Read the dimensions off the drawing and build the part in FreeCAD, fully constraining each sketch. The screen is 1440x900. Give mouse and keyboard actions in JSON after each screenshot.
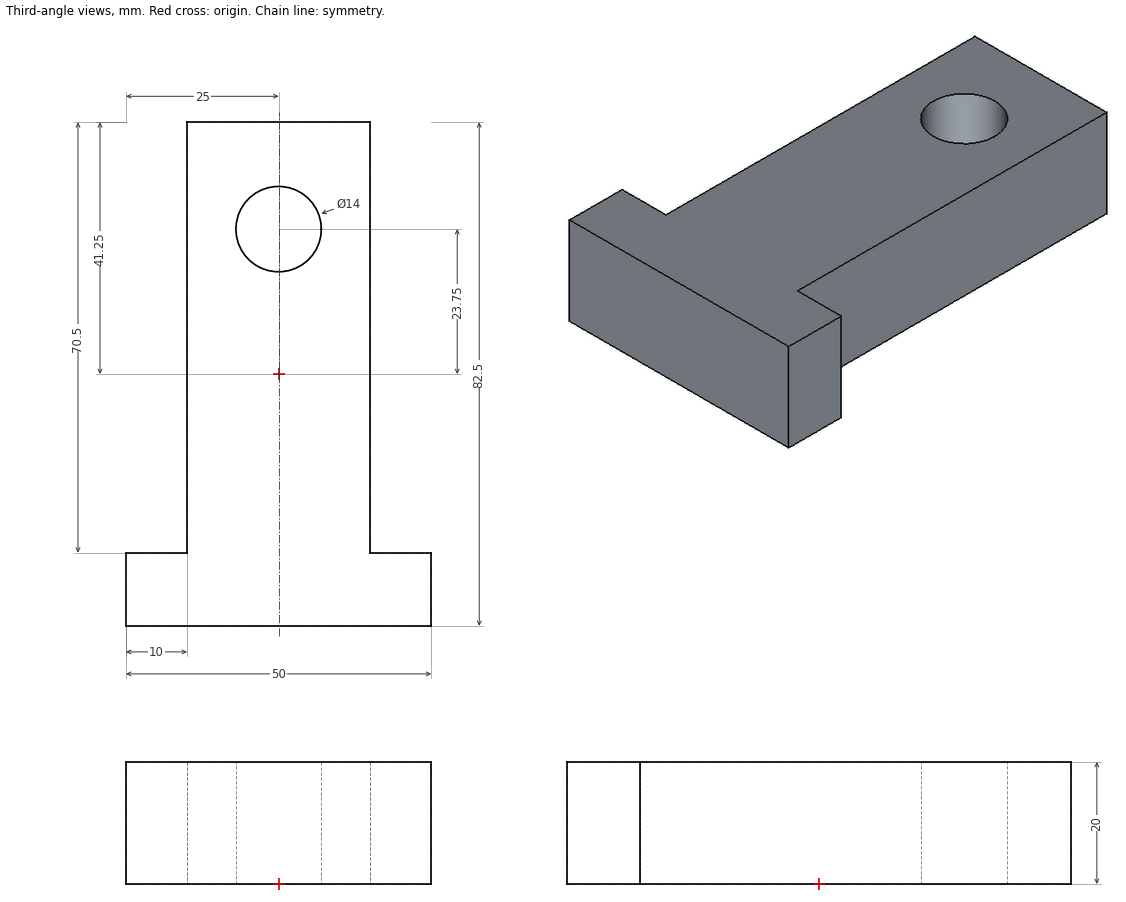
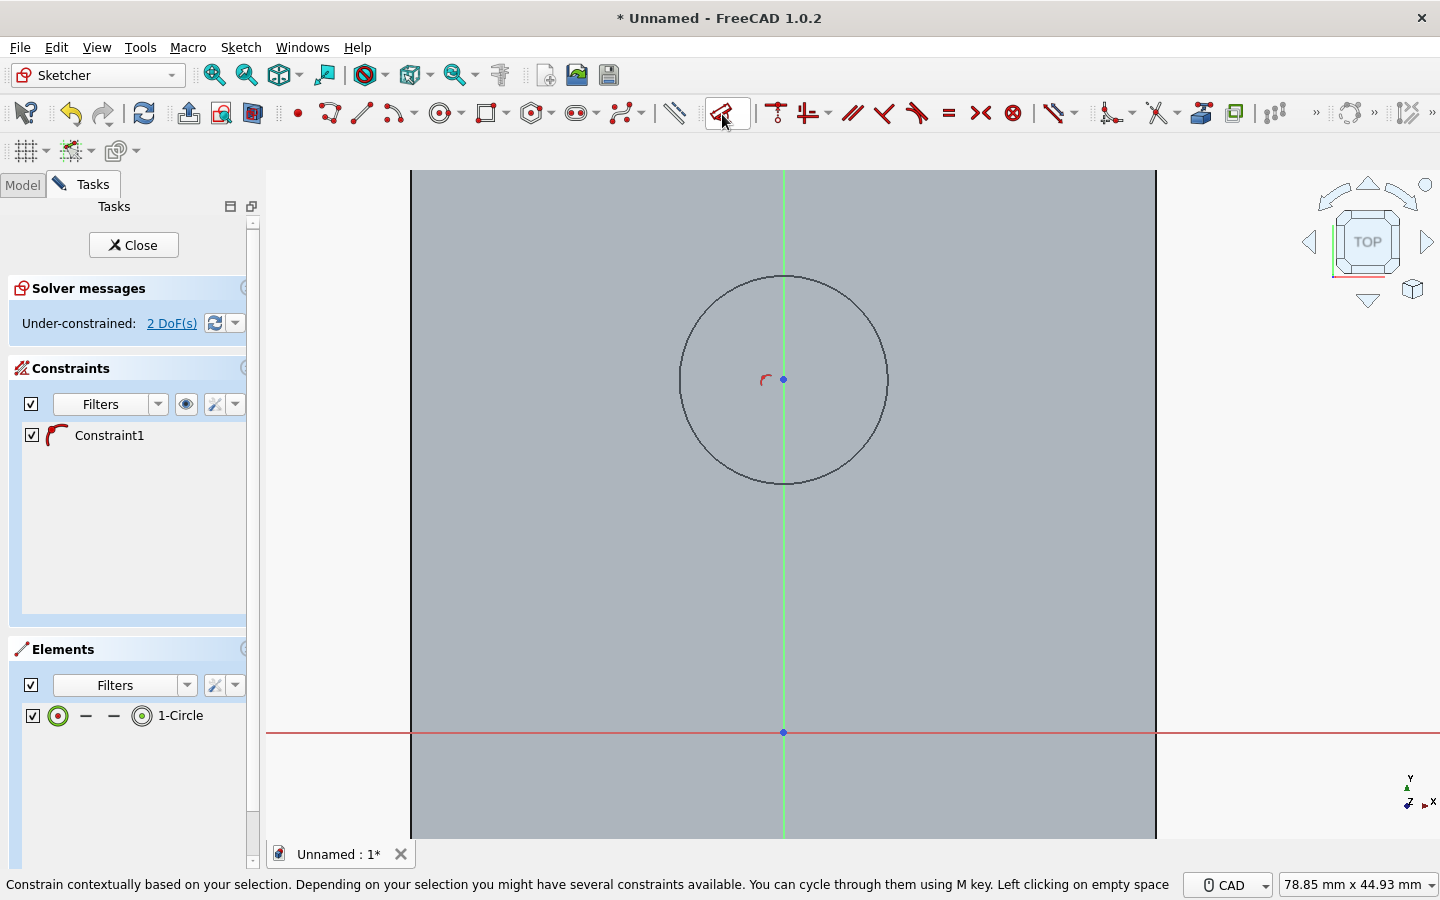
{"action": "left_click", "coordinate": [857, 306]}
{"action": "left_click", "coordinate": [880, 283]}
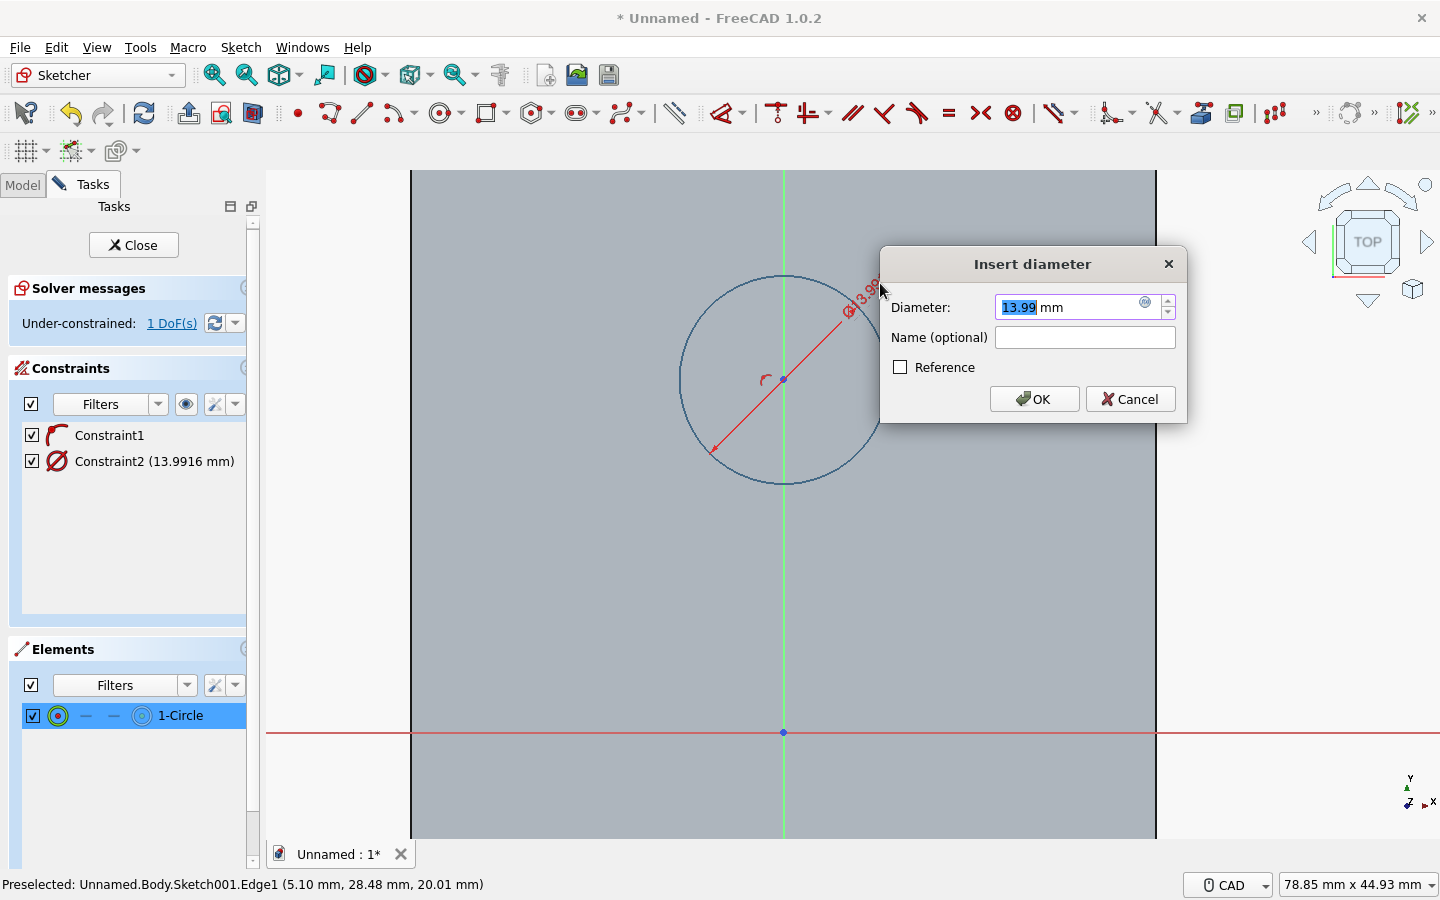
{"action": "type", "text": "14"}
{"action": "key", "text": "Return"}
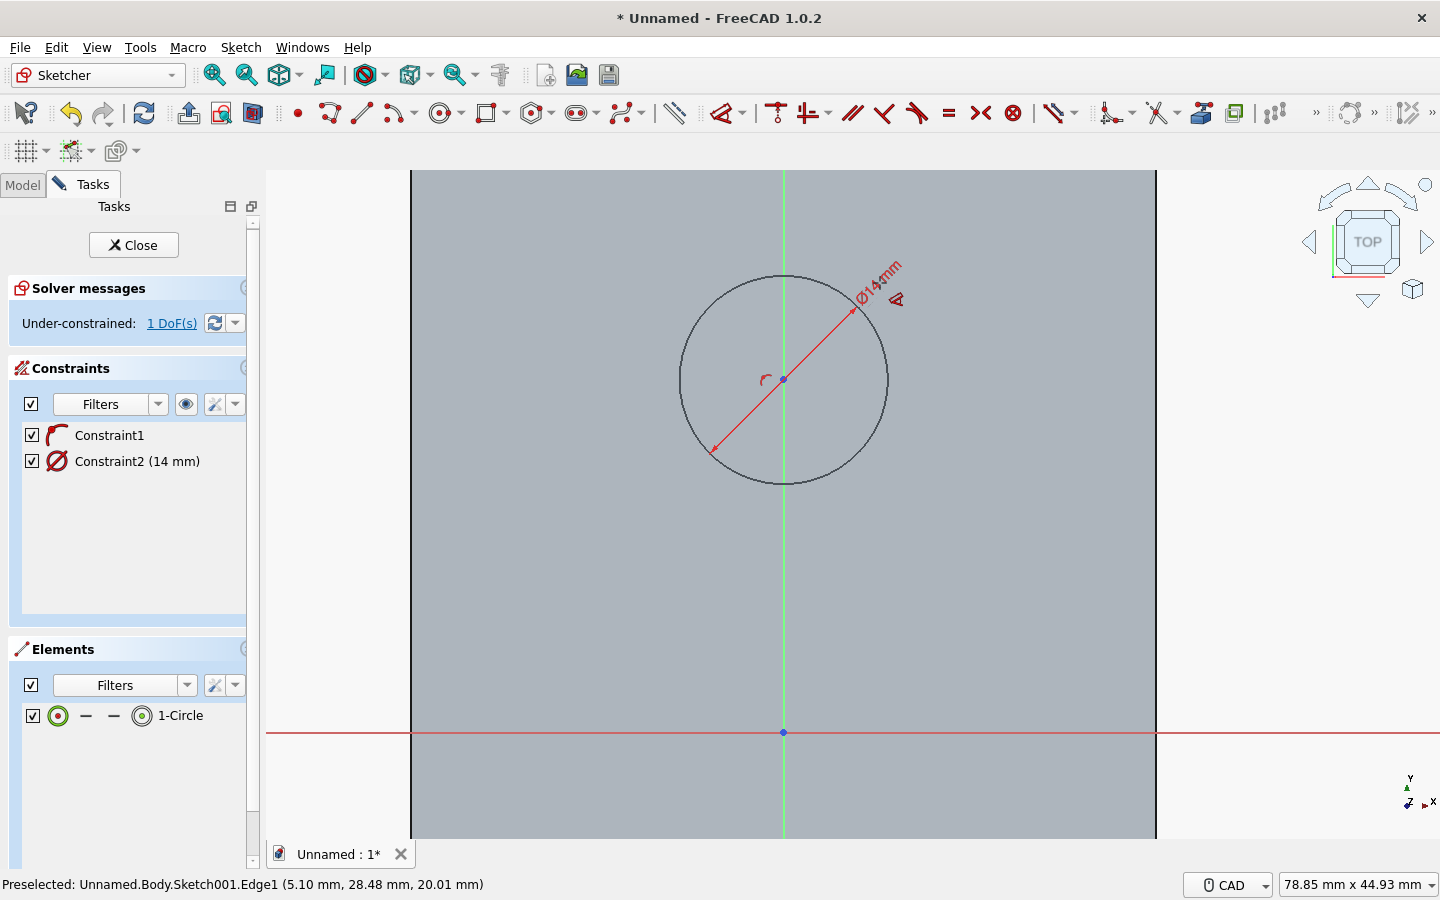
{"action": "left_click", "coordinate": [784, 380]}
{"action": "left_click", "coordinate": [818, 556]}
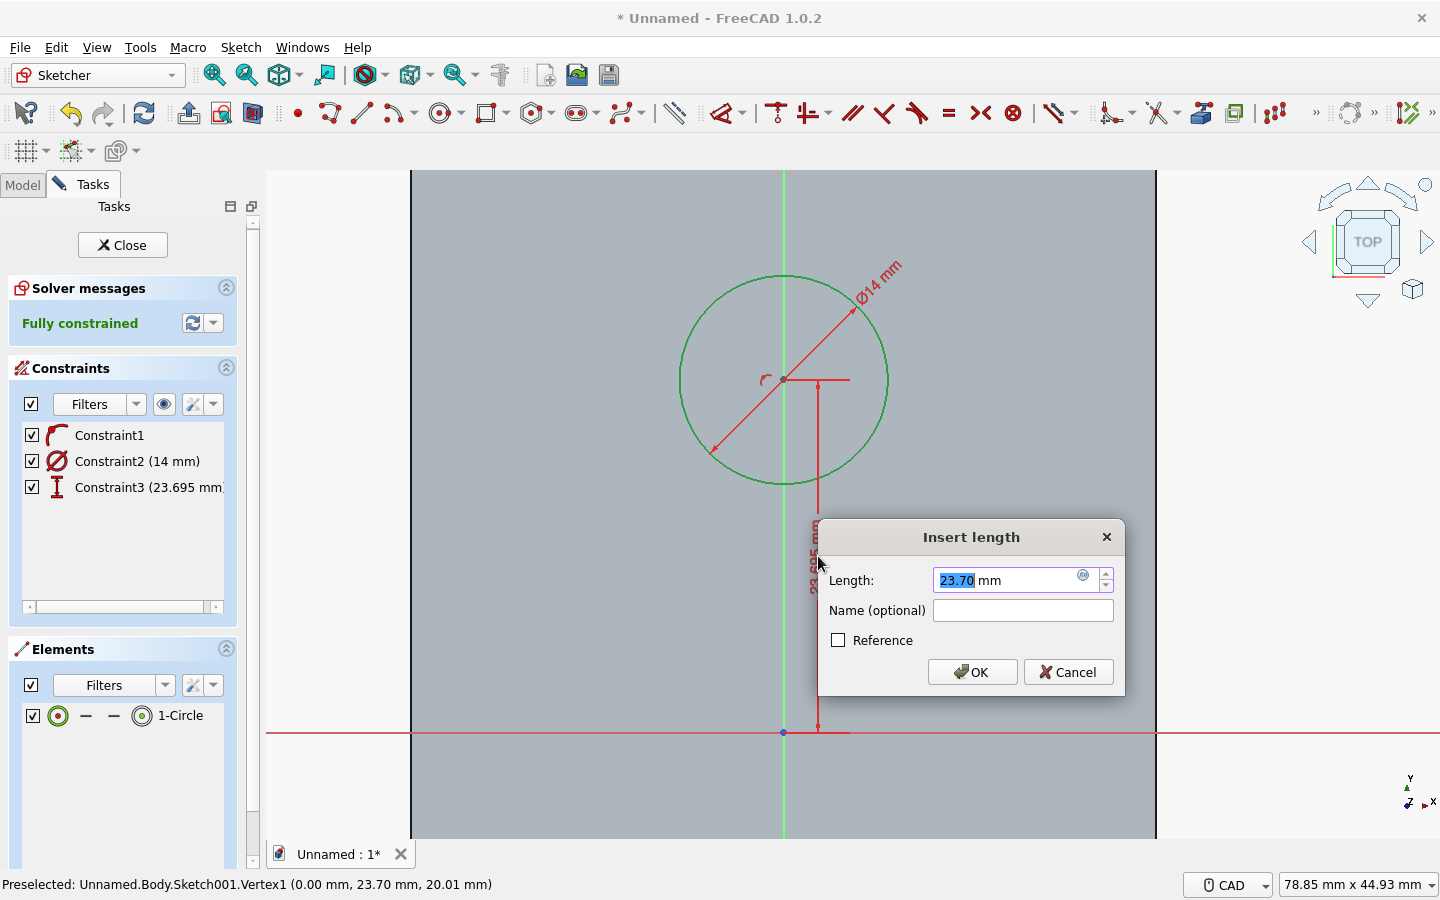
{"action": "type", "text": "23.75"}
{"action": "key", "text": "Return"}
{"action": "key", "text": "Escape"}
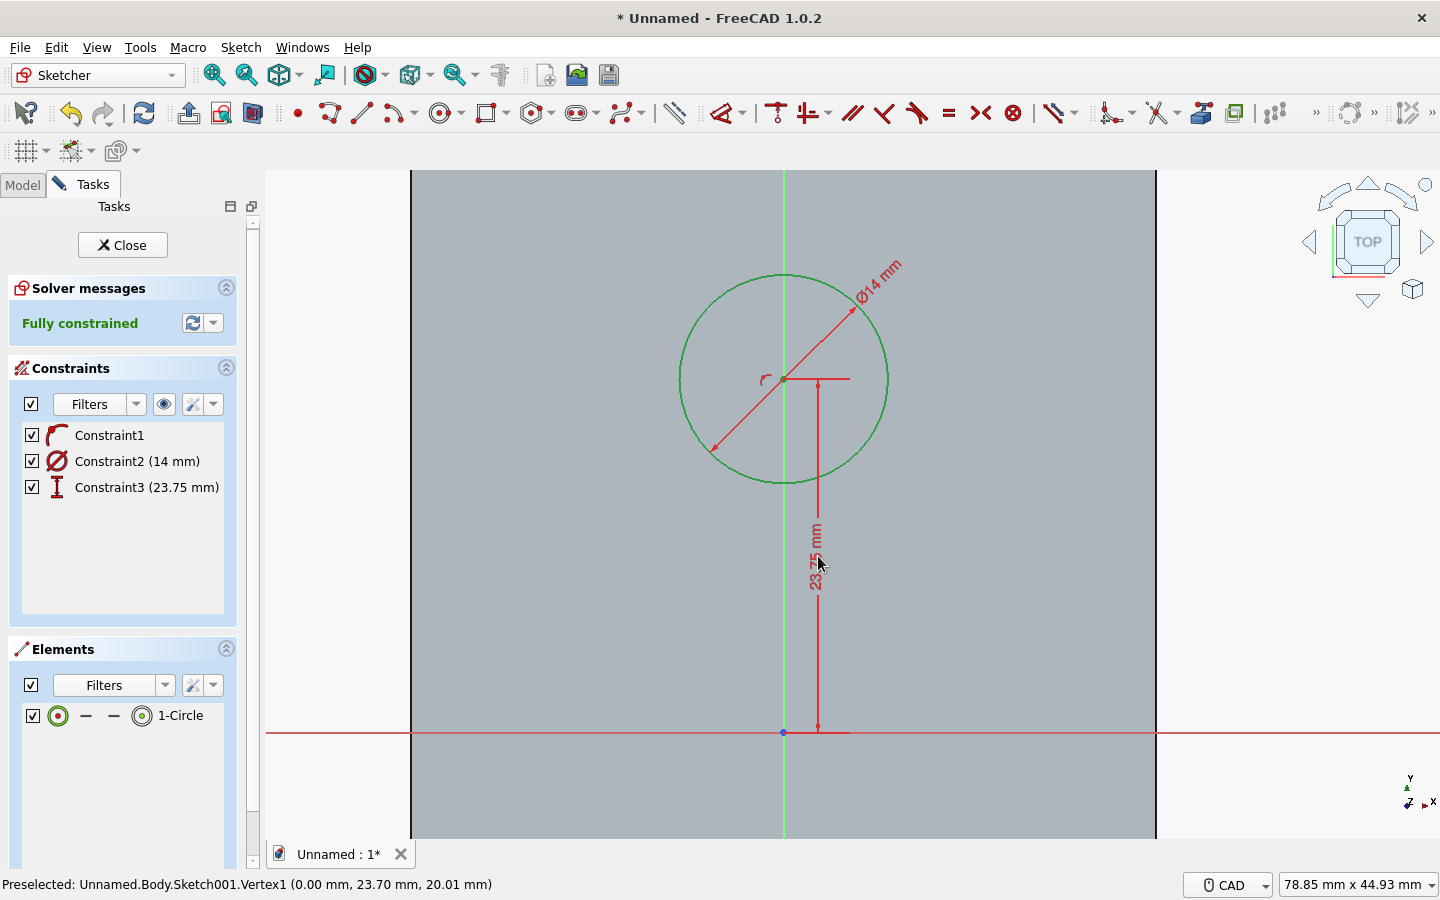
{"action": "left_click", "coordinate": [123, 245]}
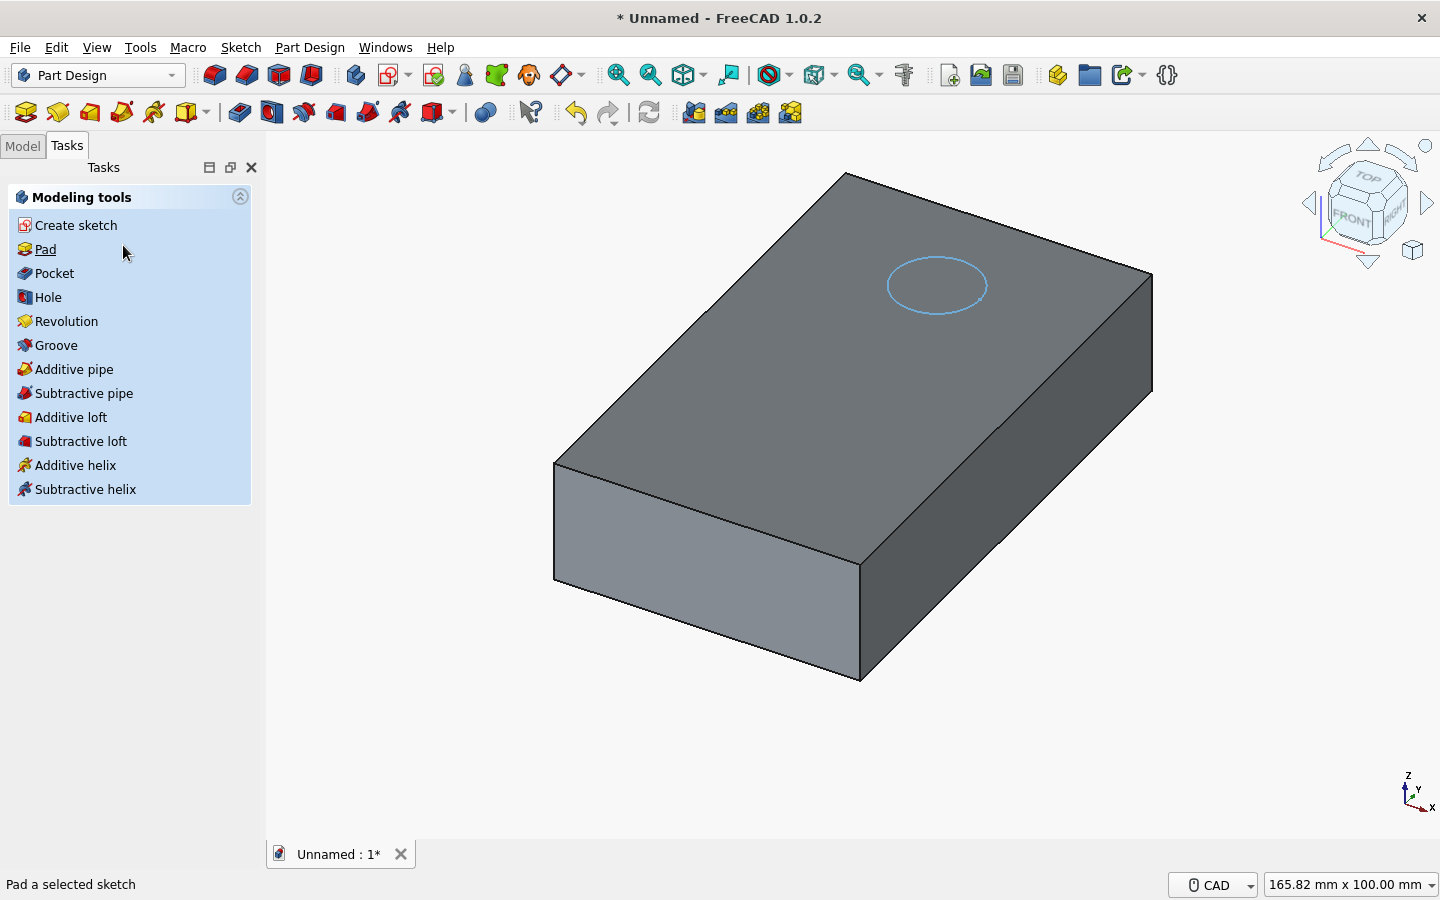
{"action": "left_click", "coordinate": [240, 112]}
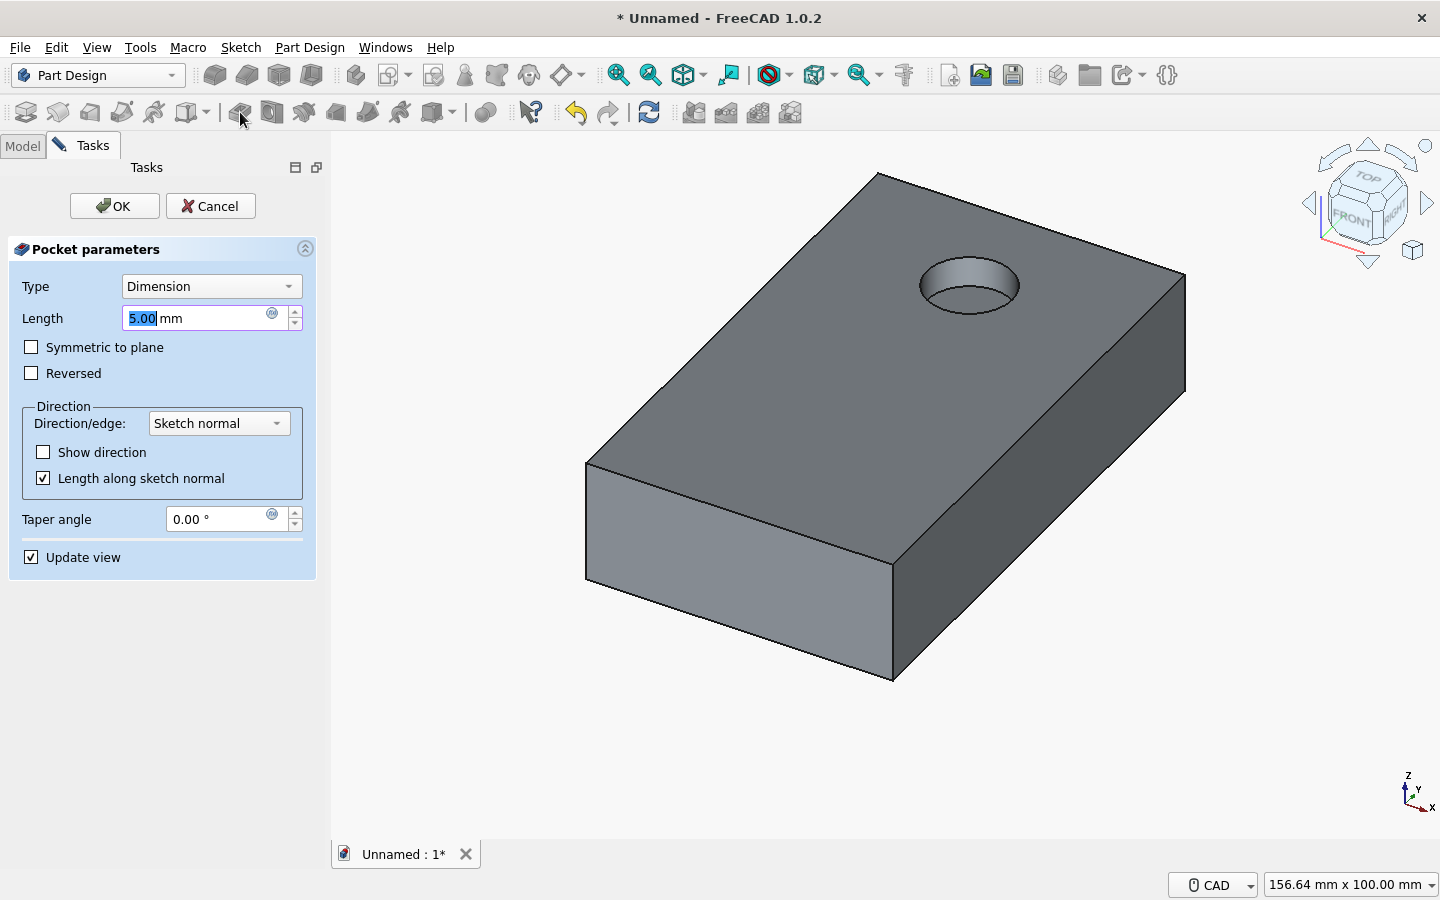
{"action": "left_click", "coordinate": [212, 286]}